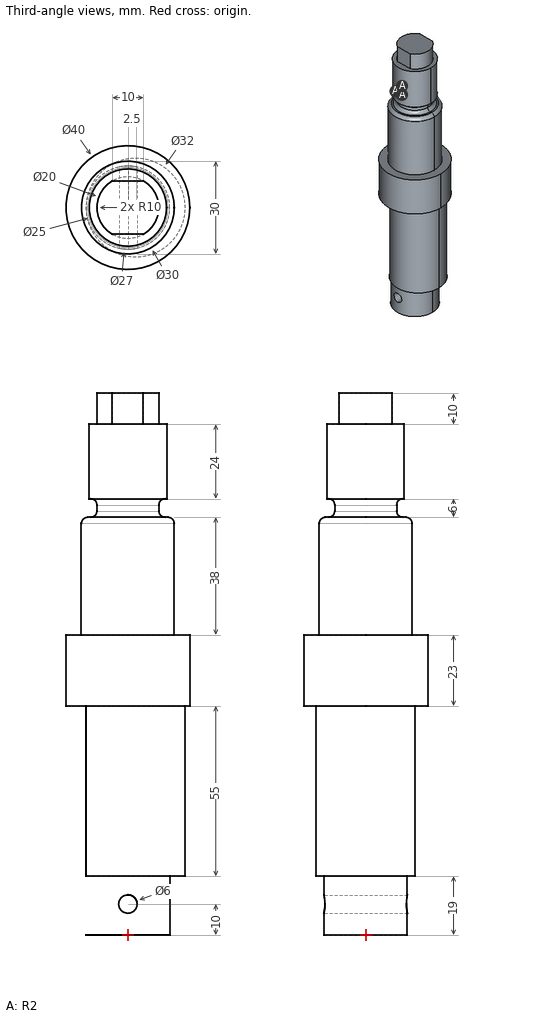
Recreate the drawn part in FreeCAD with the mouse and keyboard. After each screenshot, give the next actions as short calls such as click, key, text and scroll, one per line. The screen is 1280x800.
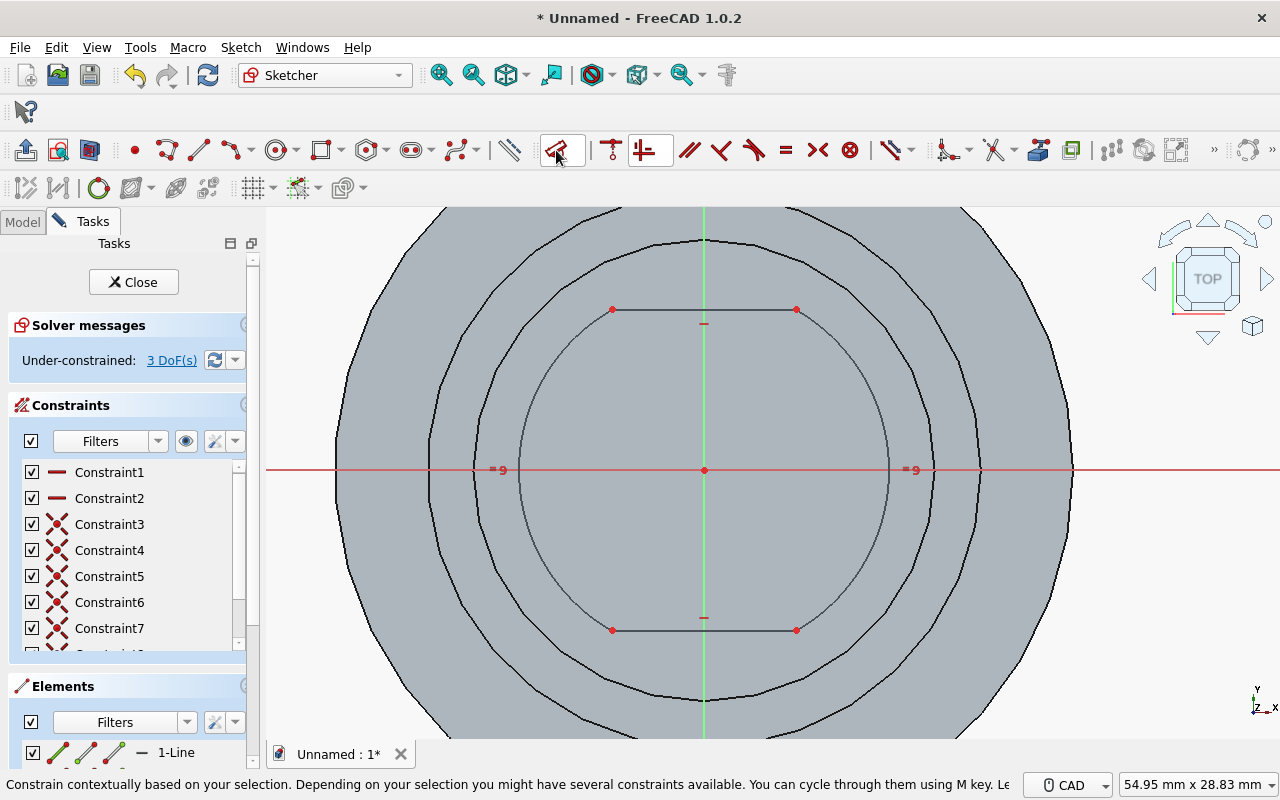
click(535, 395)
click(506, 382)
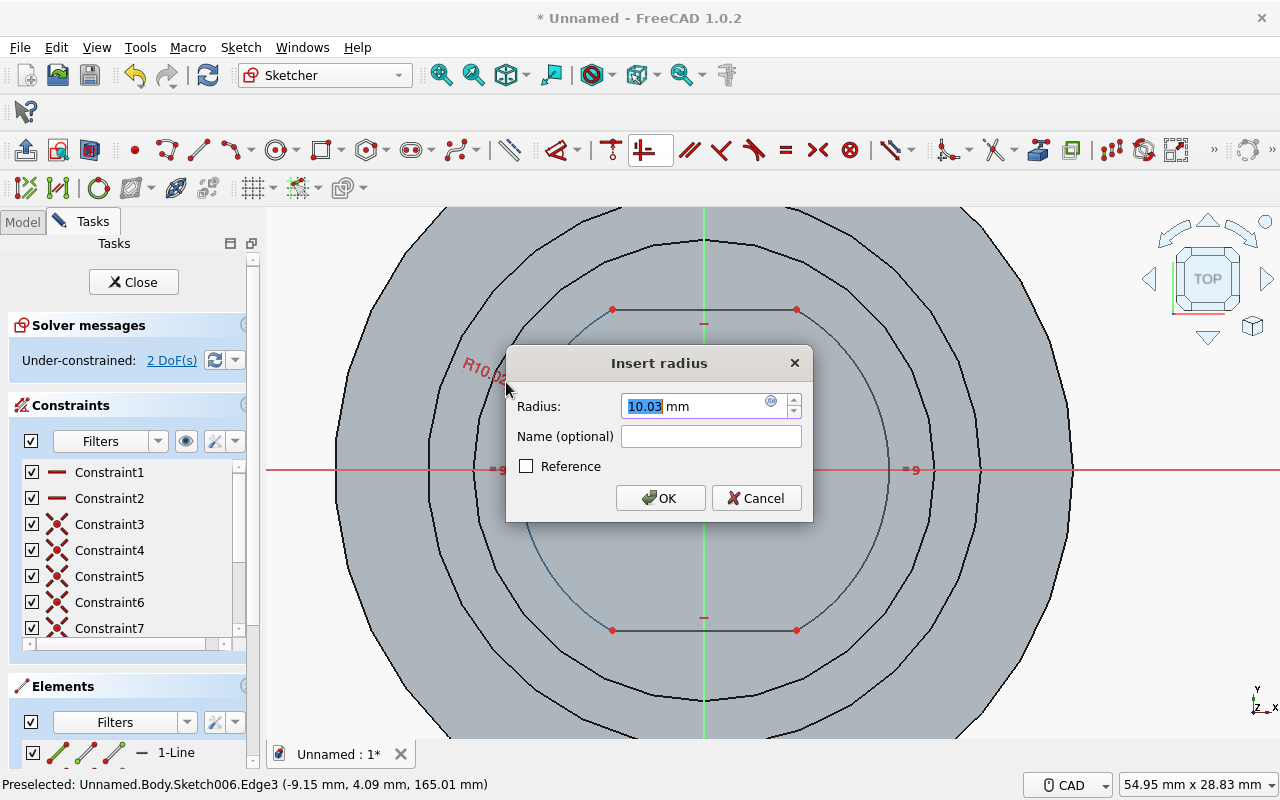
text(10)
key(Return)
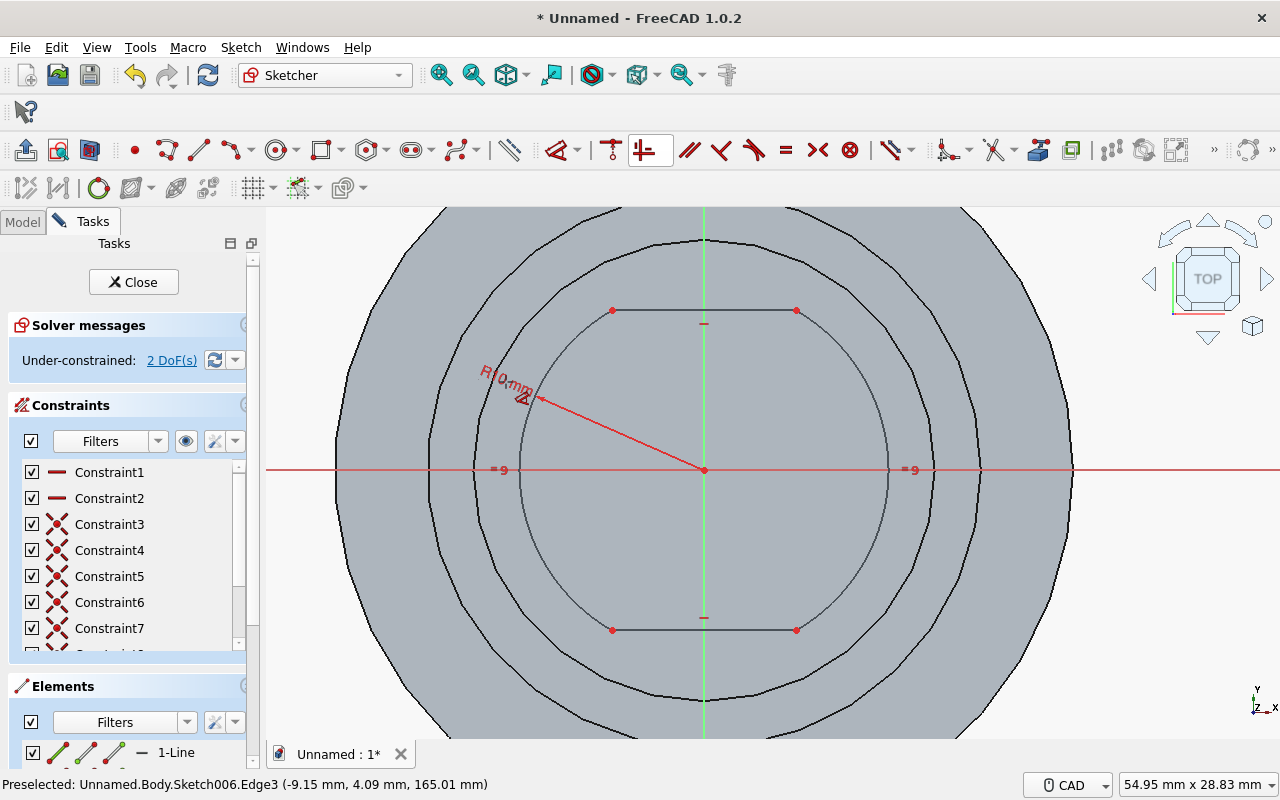
click(741, 310)
click(662, 276)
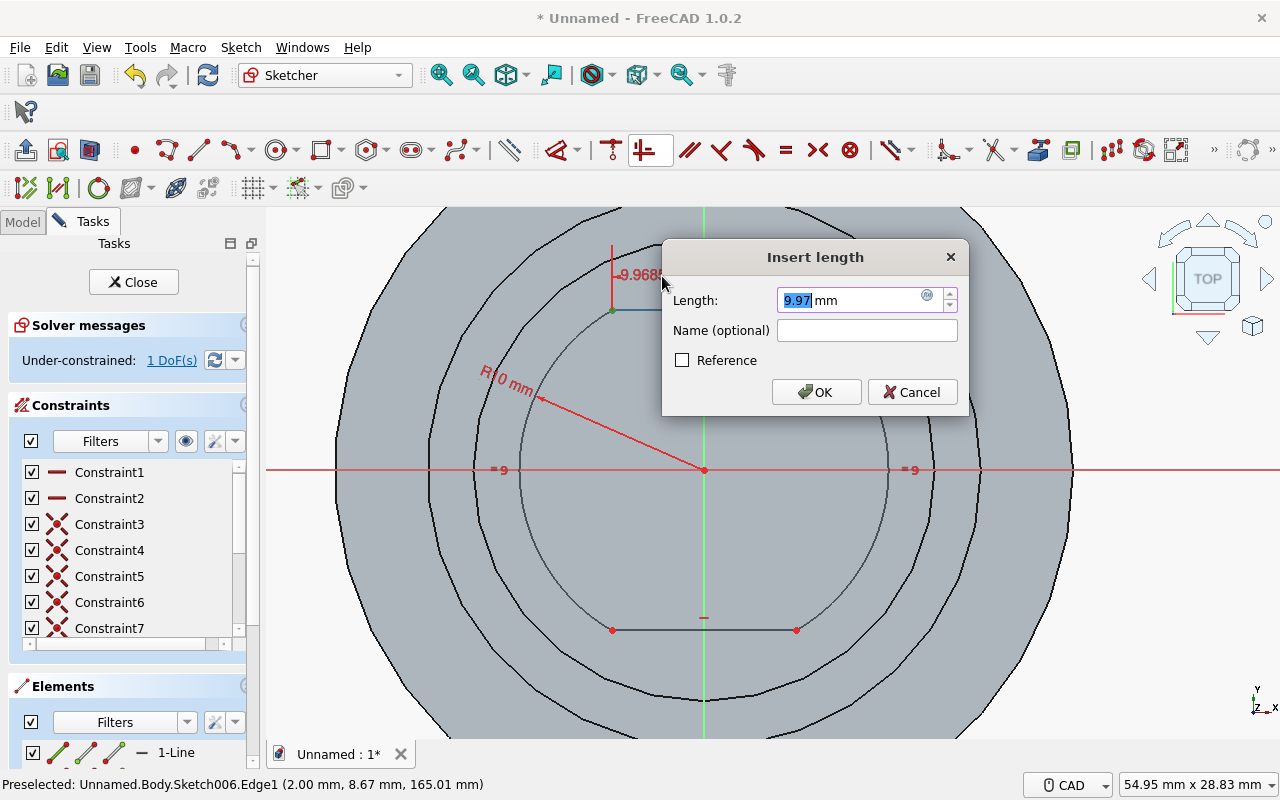
text(10)
key(Return)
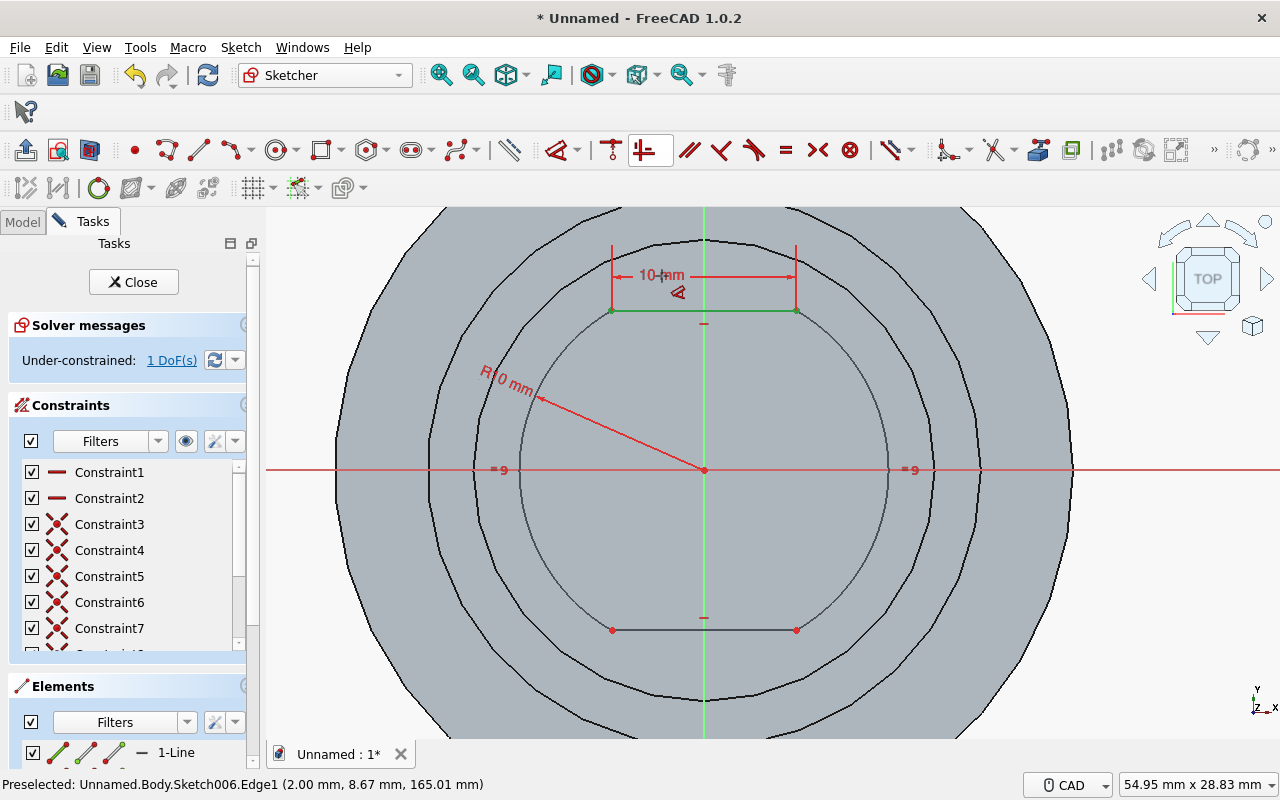
click(667, 630)
click(662, 664)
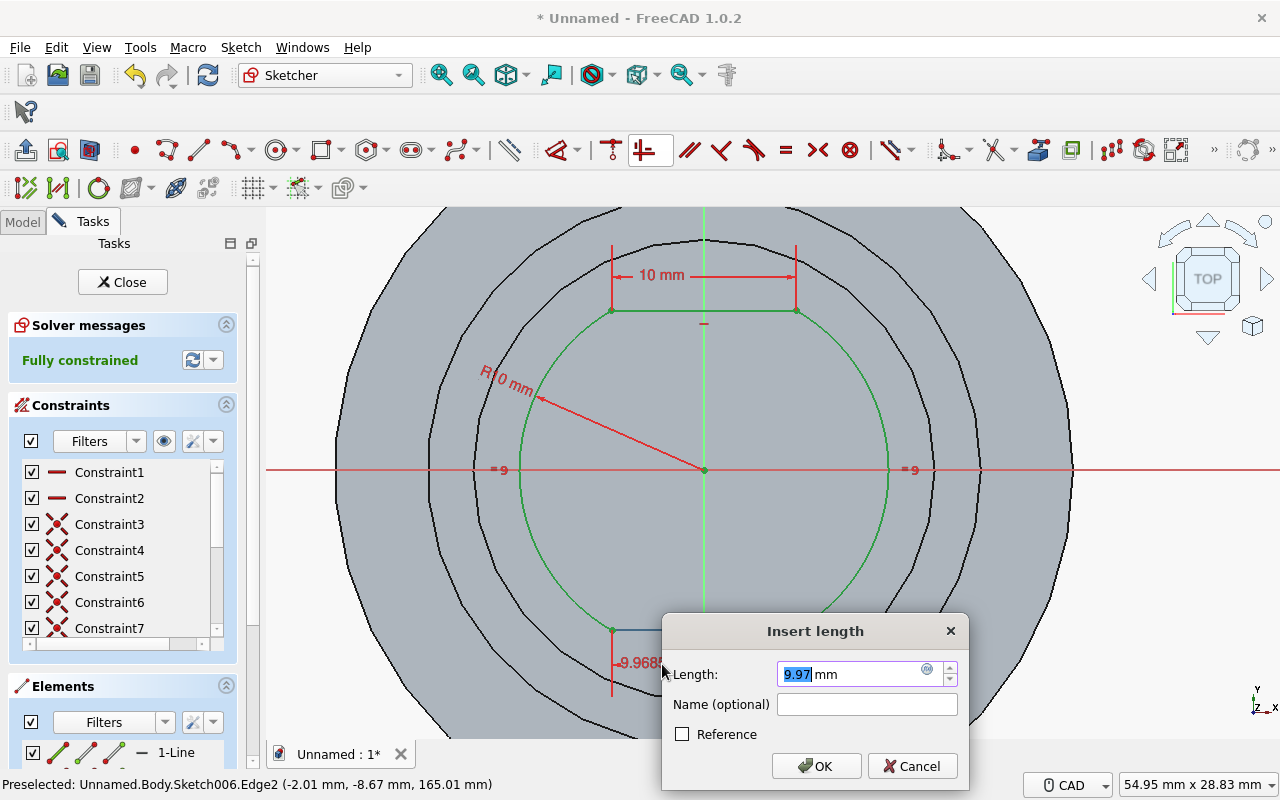
text(10)
key(Return)
key(Escape)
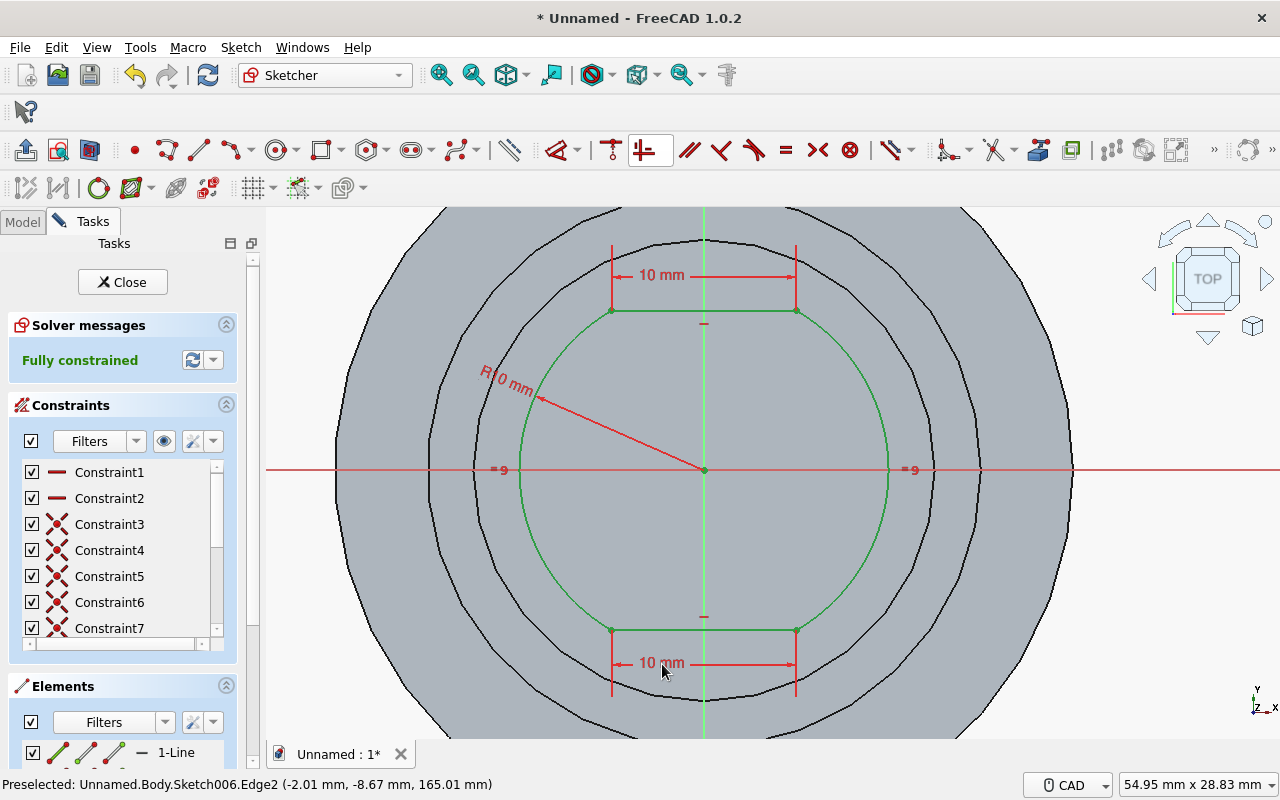
click(123, 282)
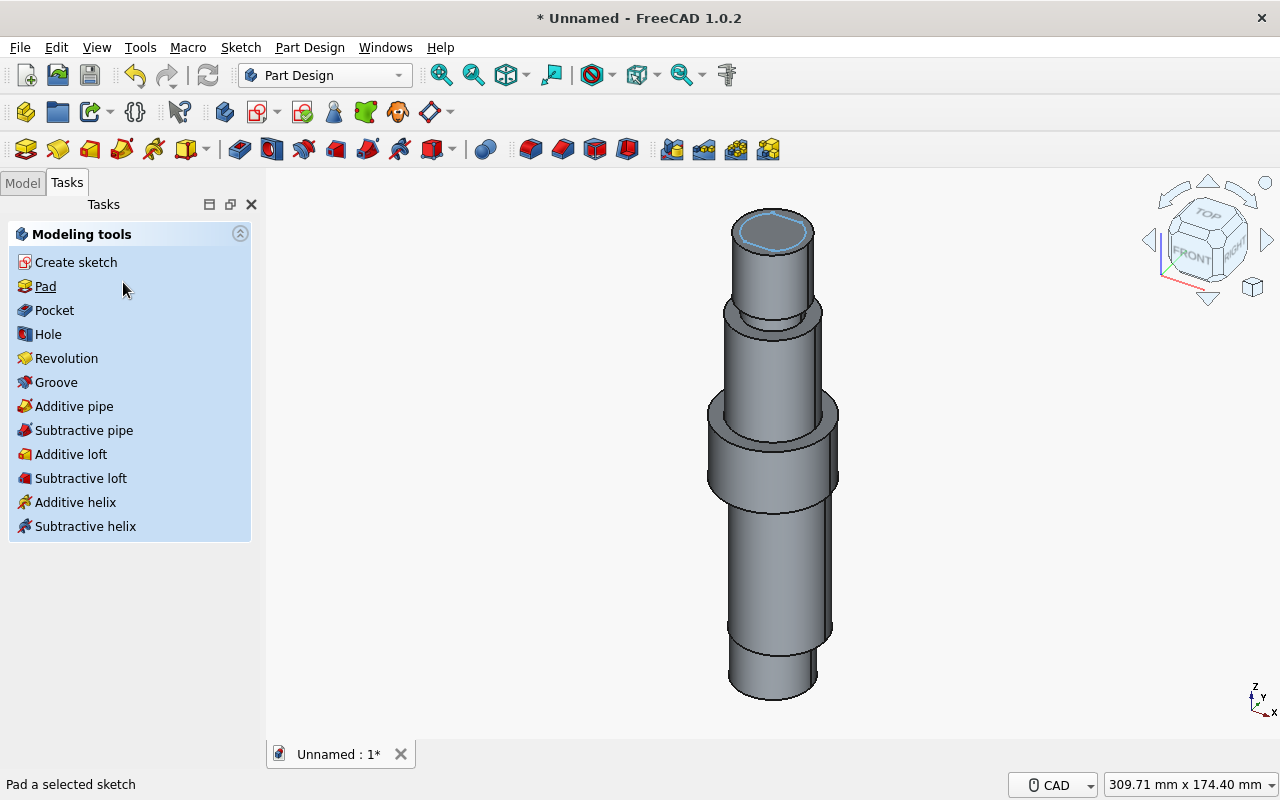
click(26, 150)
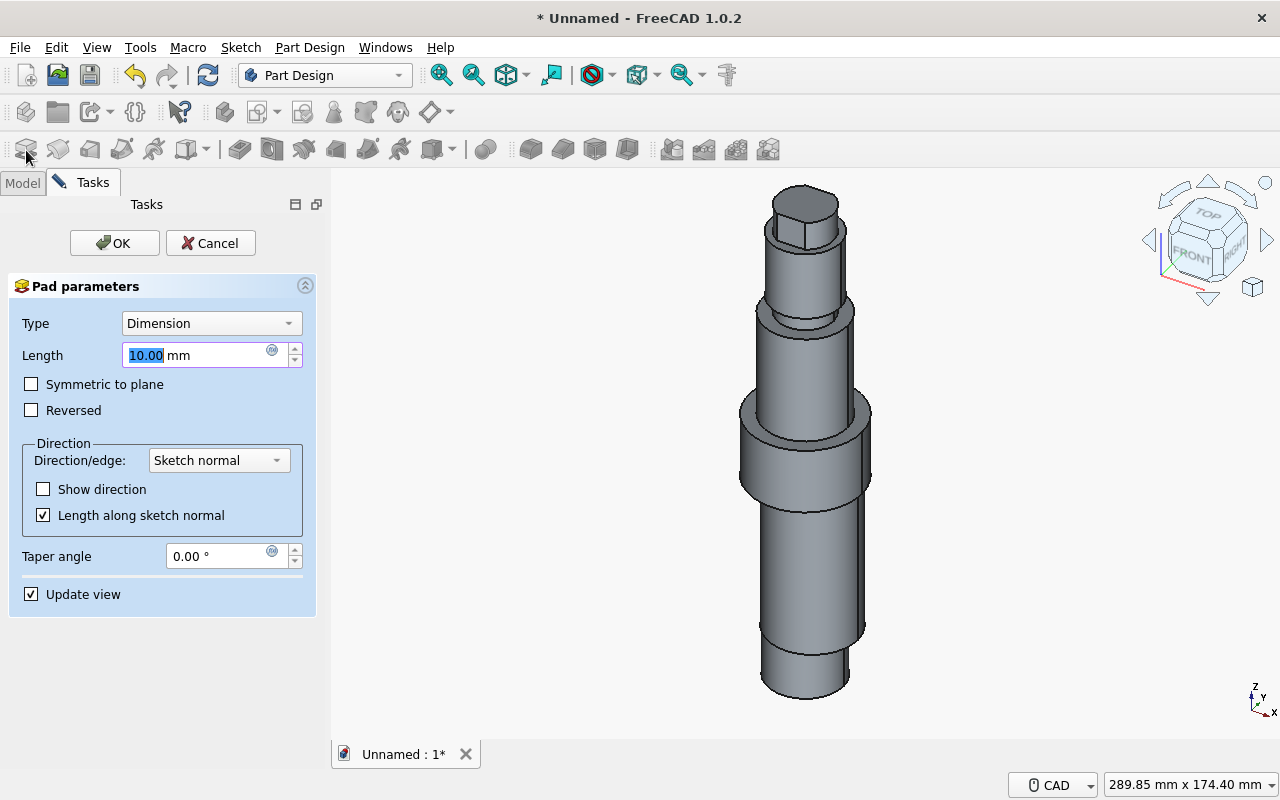
text(10)
key(Tab)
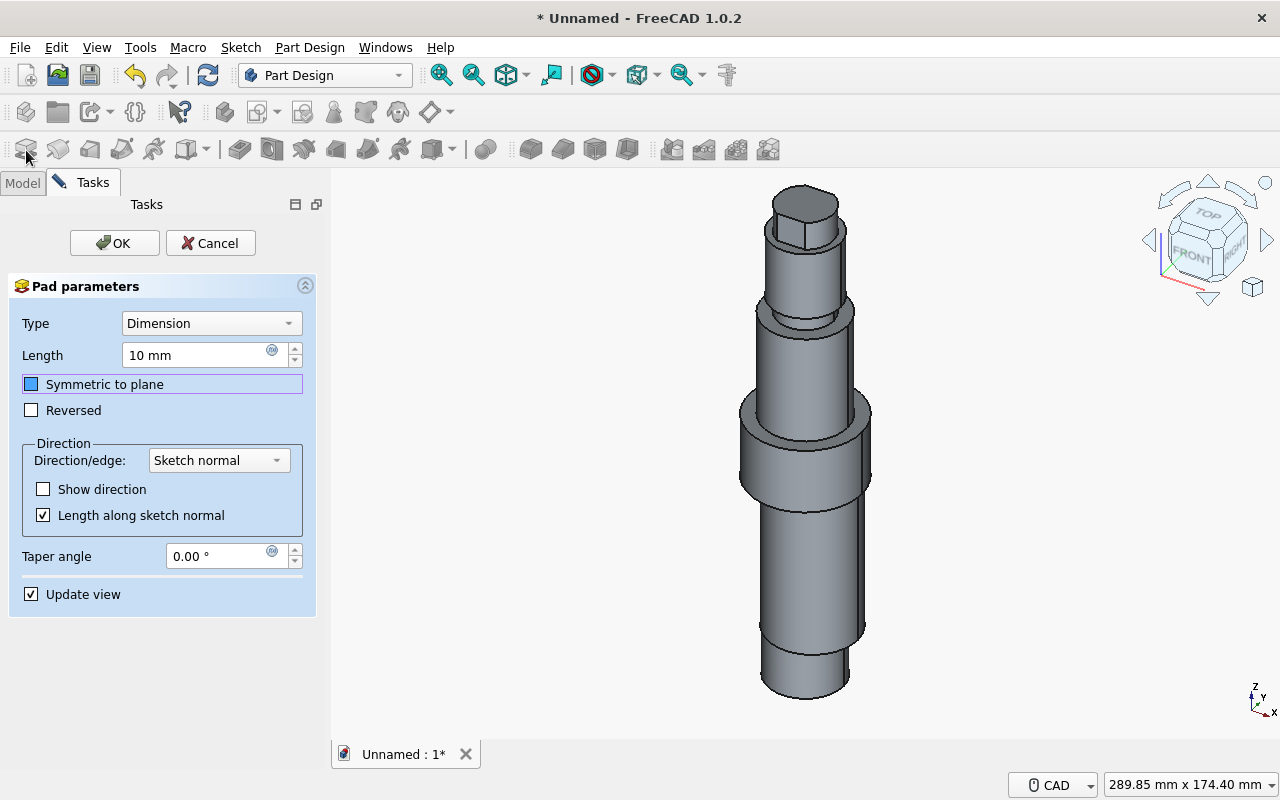
click(115, 243)